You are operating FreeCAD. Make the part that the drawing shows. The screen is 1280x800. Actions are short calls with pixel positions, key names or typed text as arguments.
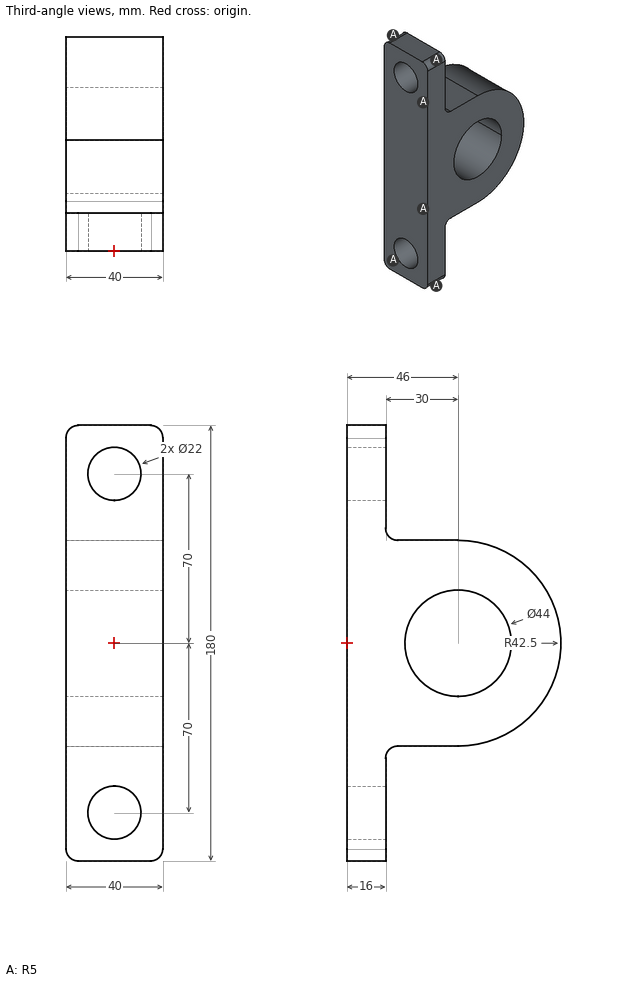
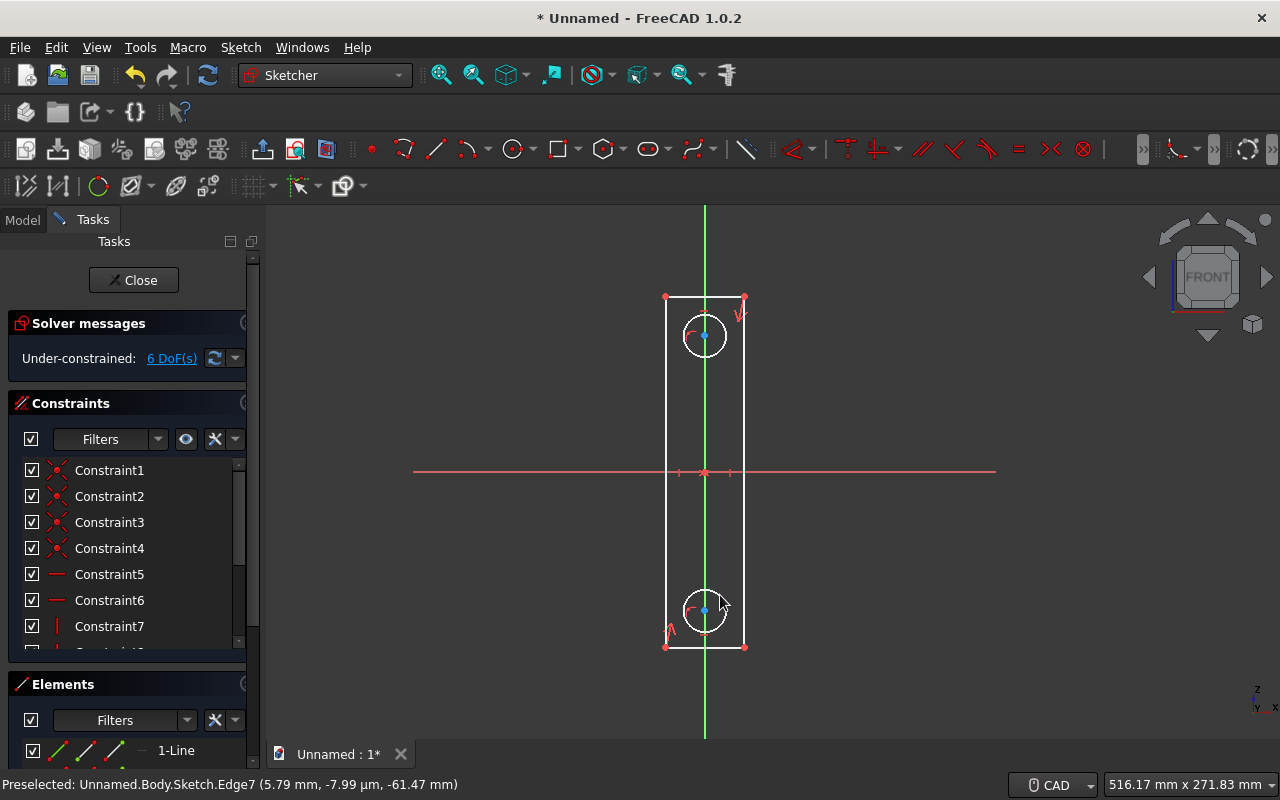
click(720, 321)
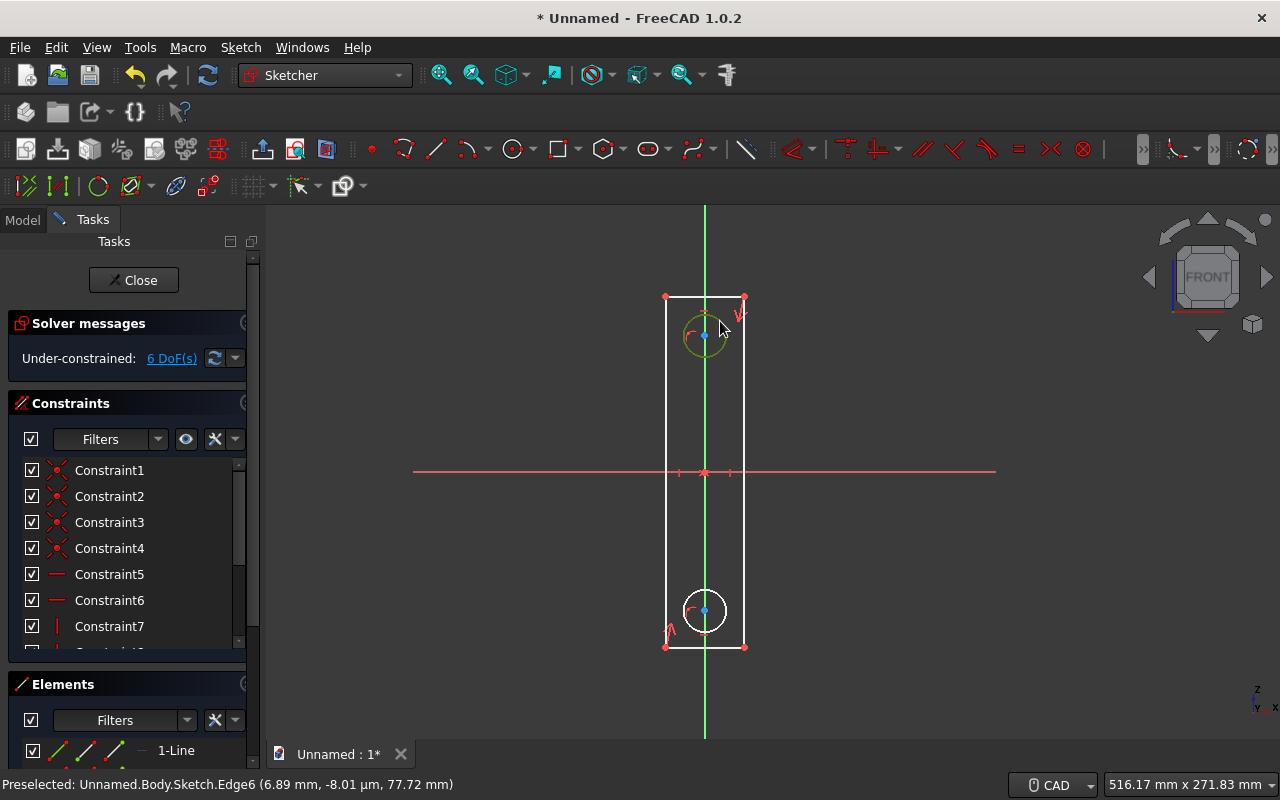
click(720, 596)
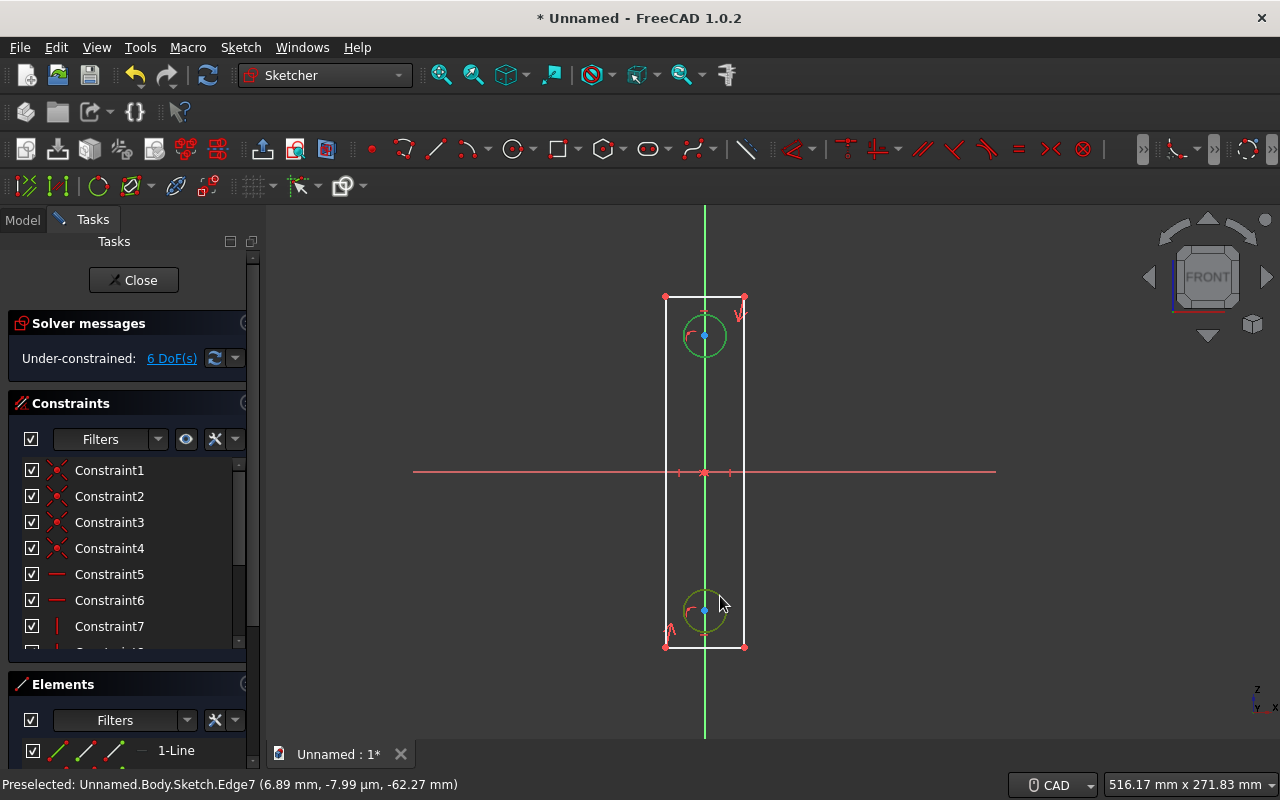
click(1020, 150)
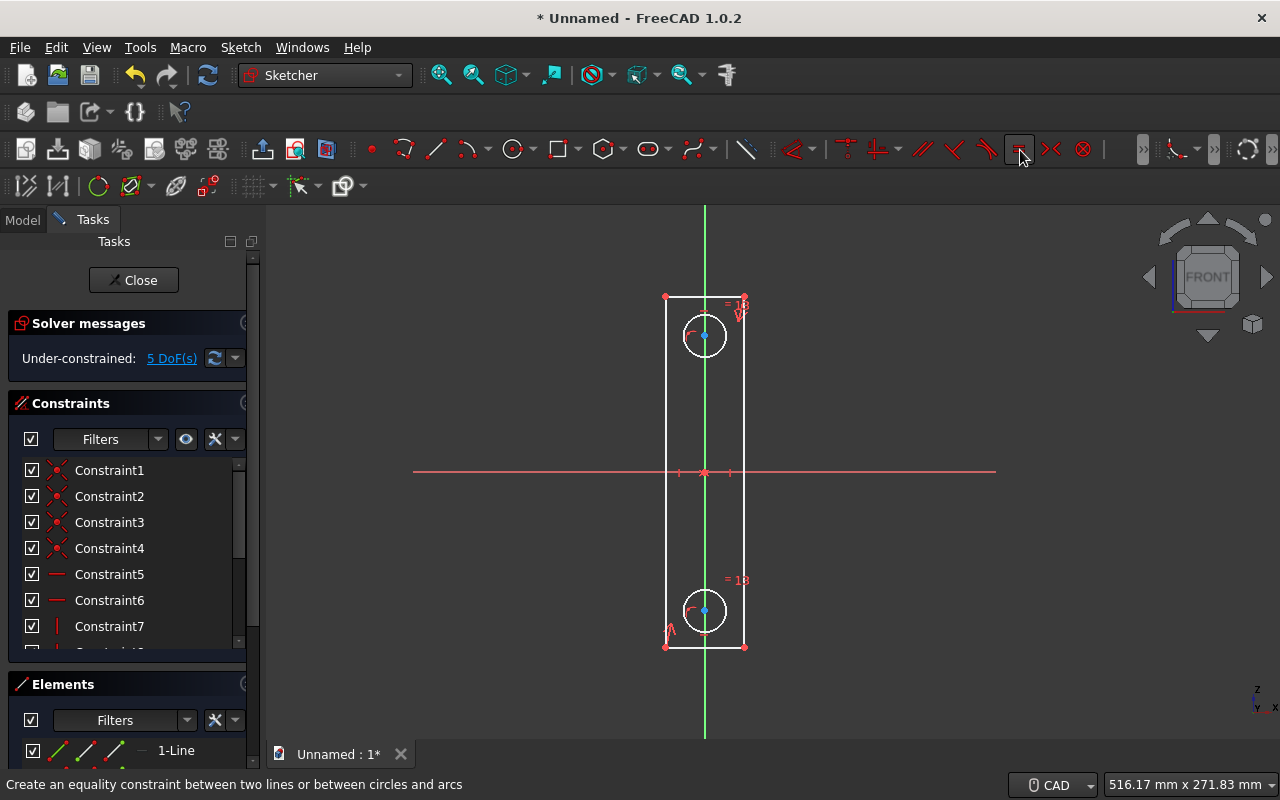
click(720, 321)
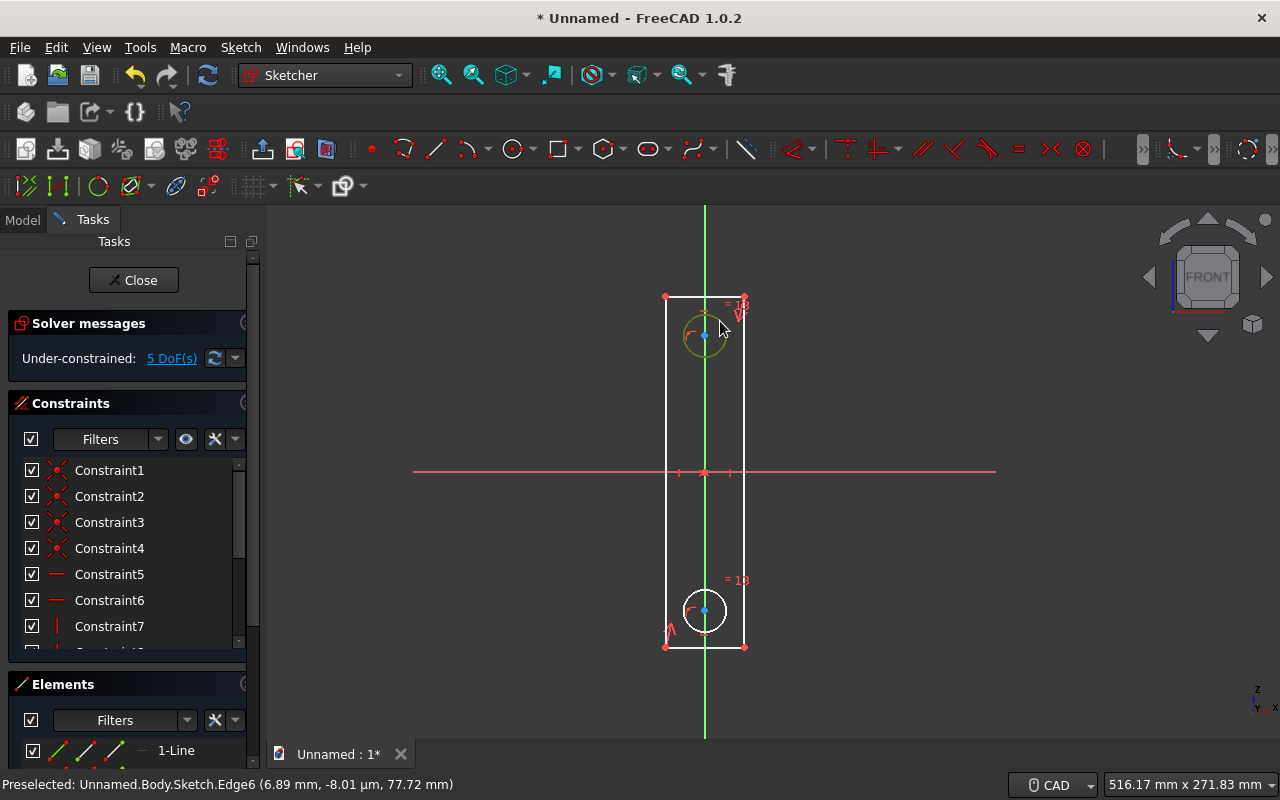
key(k)
key(o)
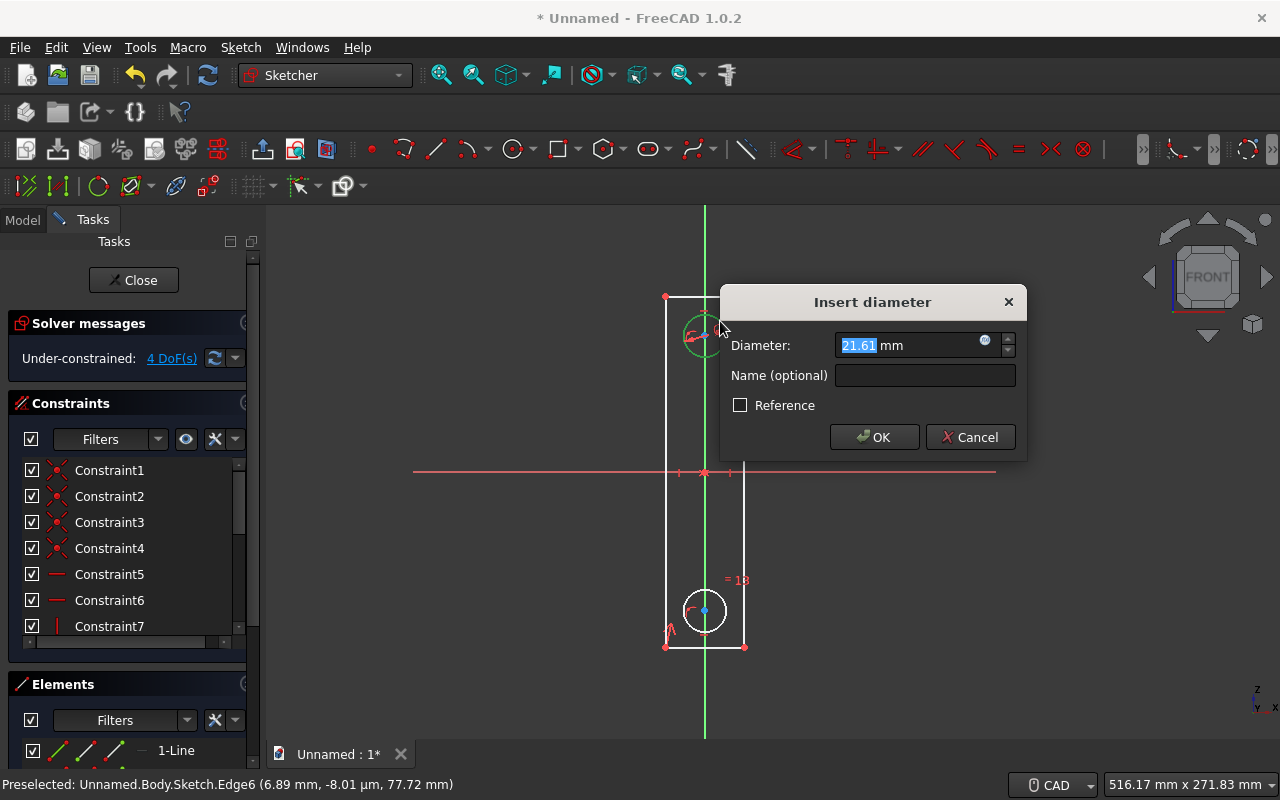
text(22)
key(Return)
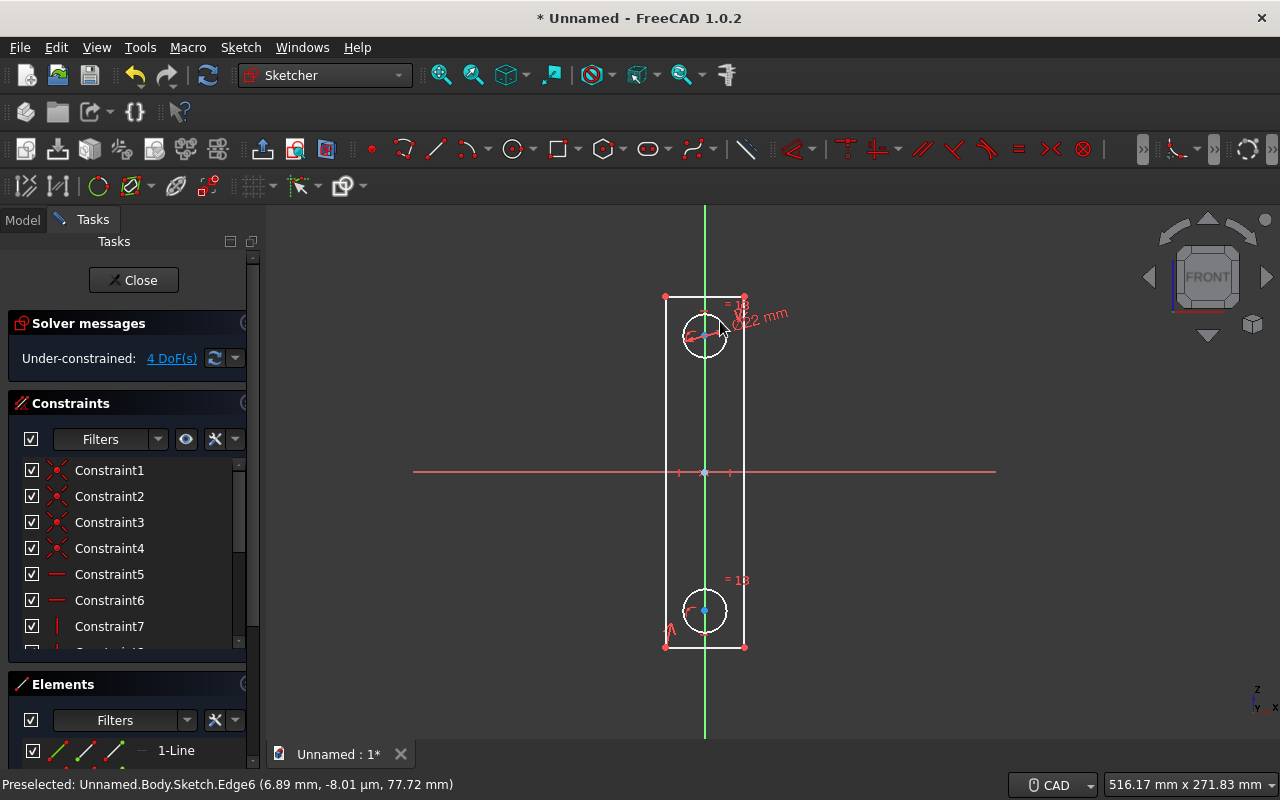
click(689, 648)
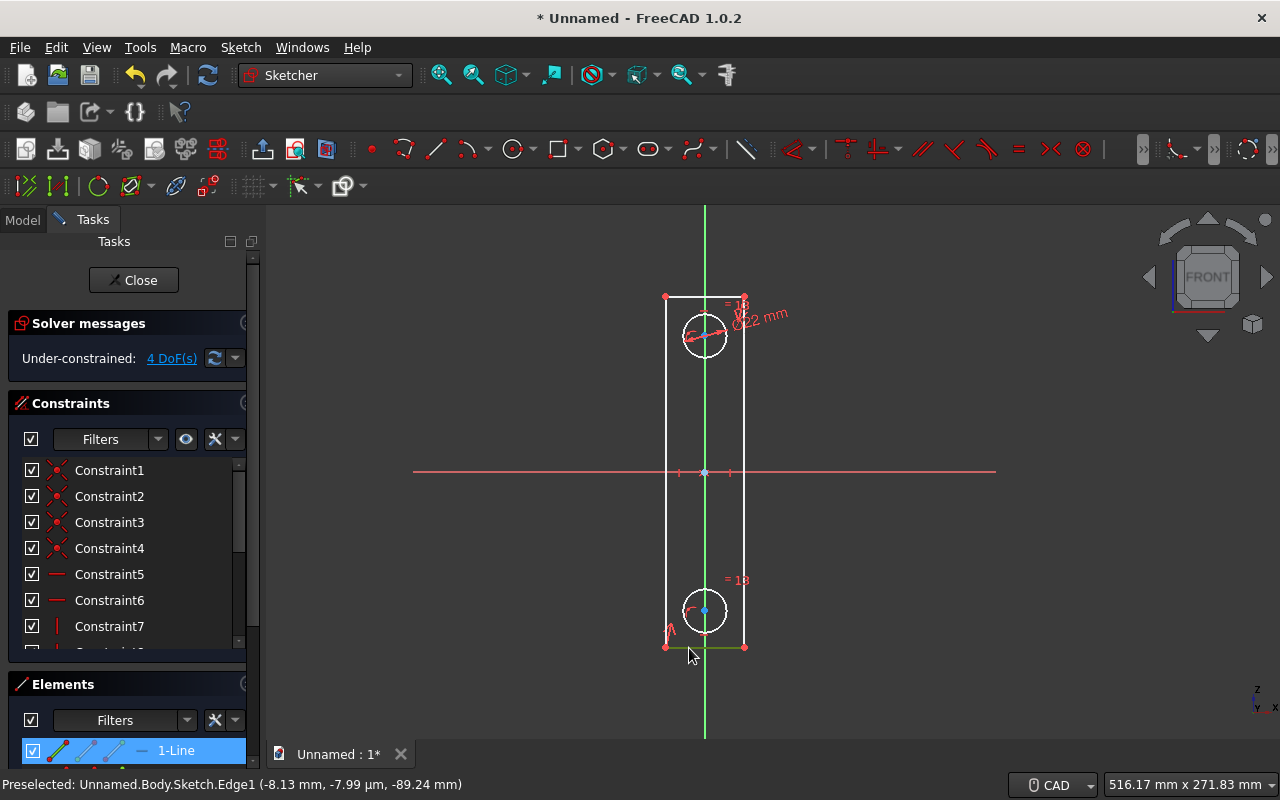
key(l)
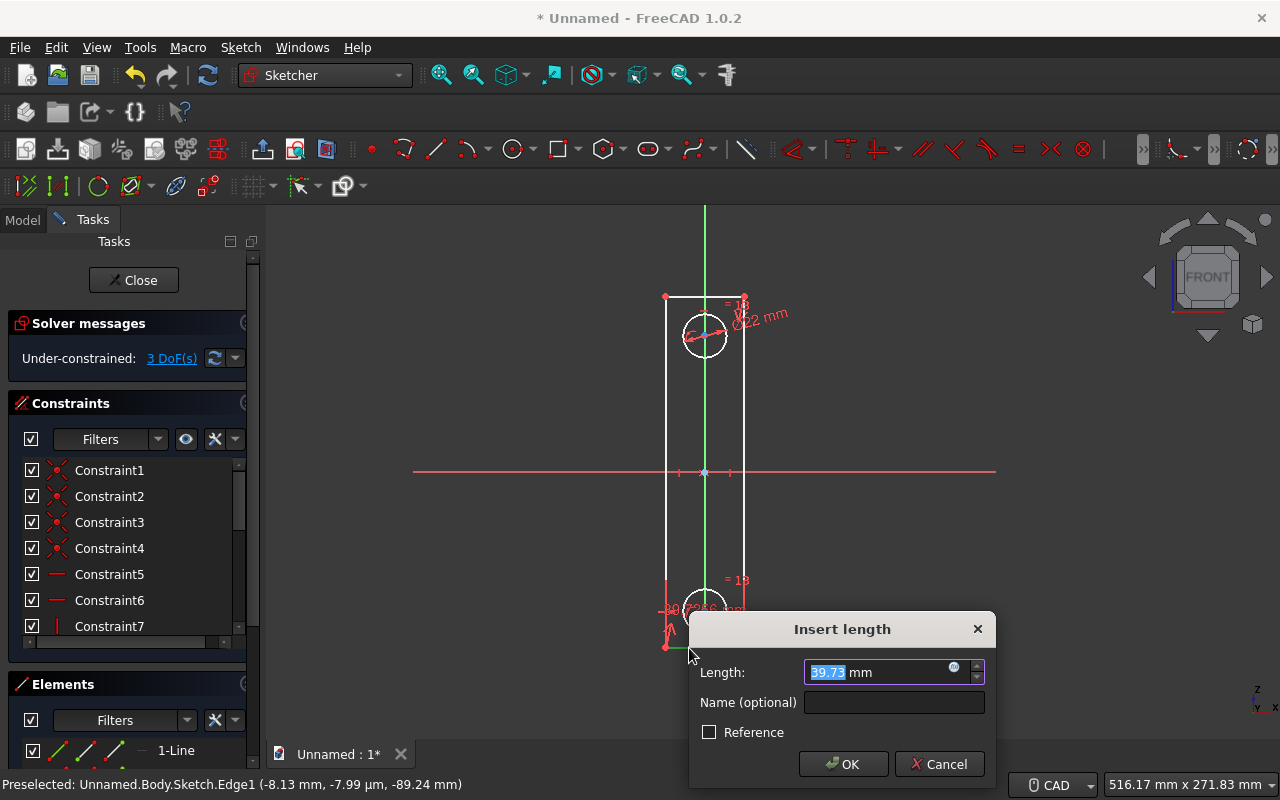
text(40)
key(Return)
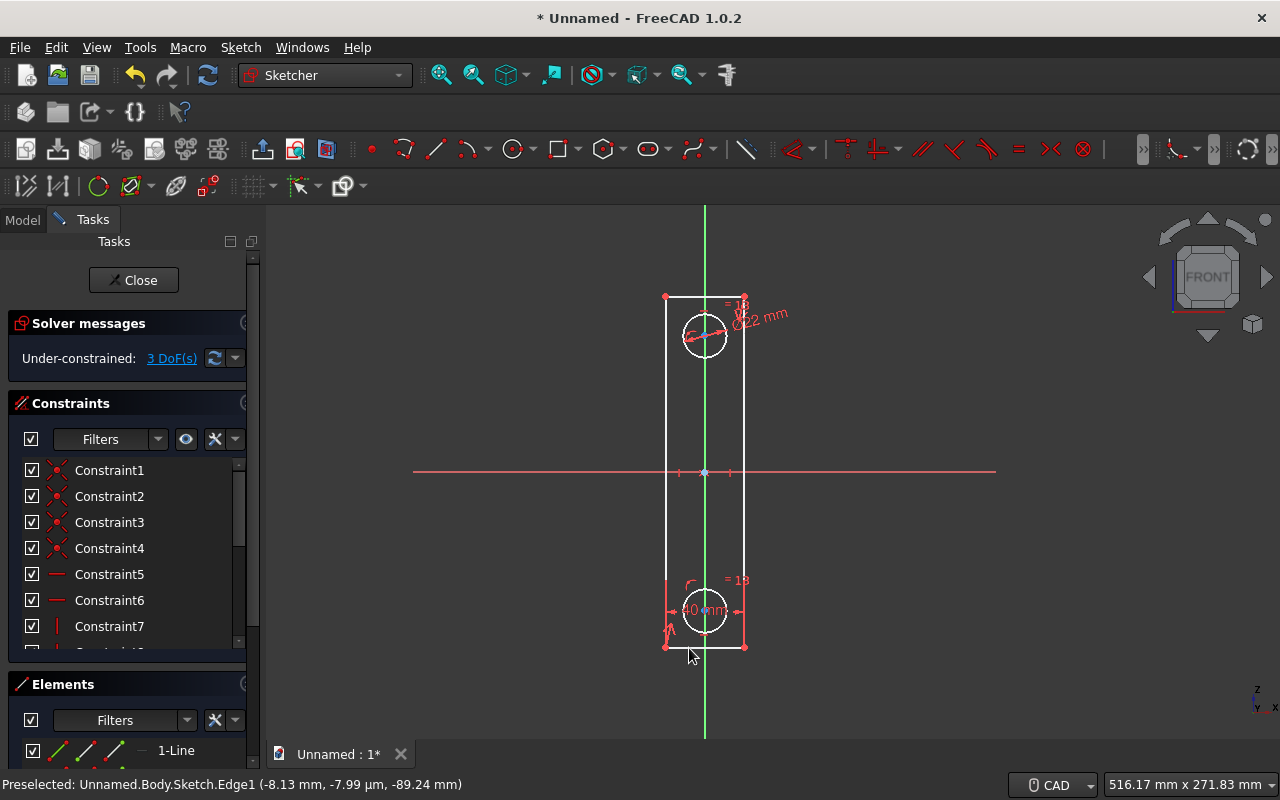
click(705, 336)